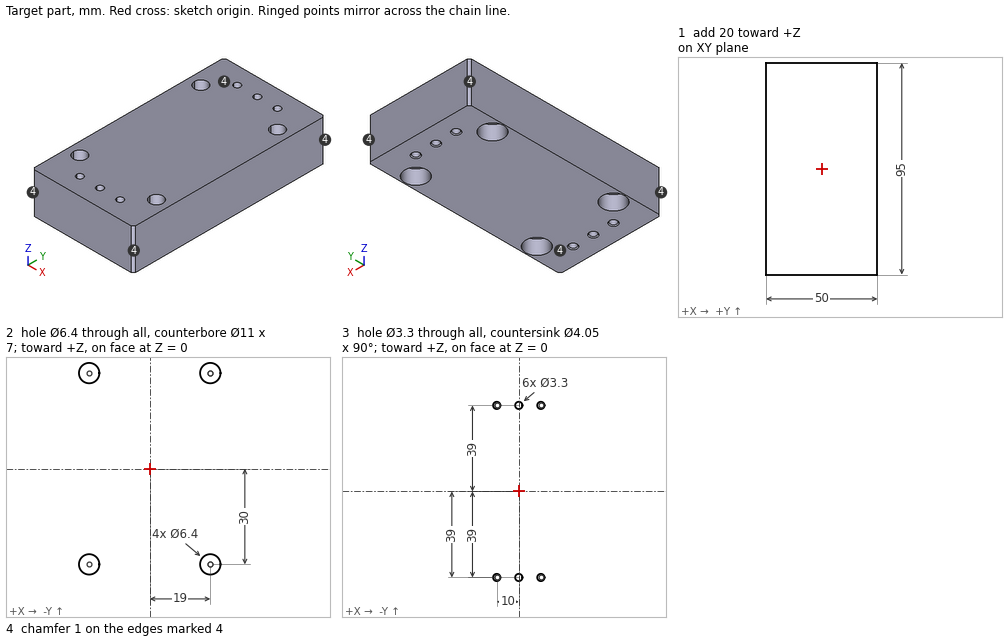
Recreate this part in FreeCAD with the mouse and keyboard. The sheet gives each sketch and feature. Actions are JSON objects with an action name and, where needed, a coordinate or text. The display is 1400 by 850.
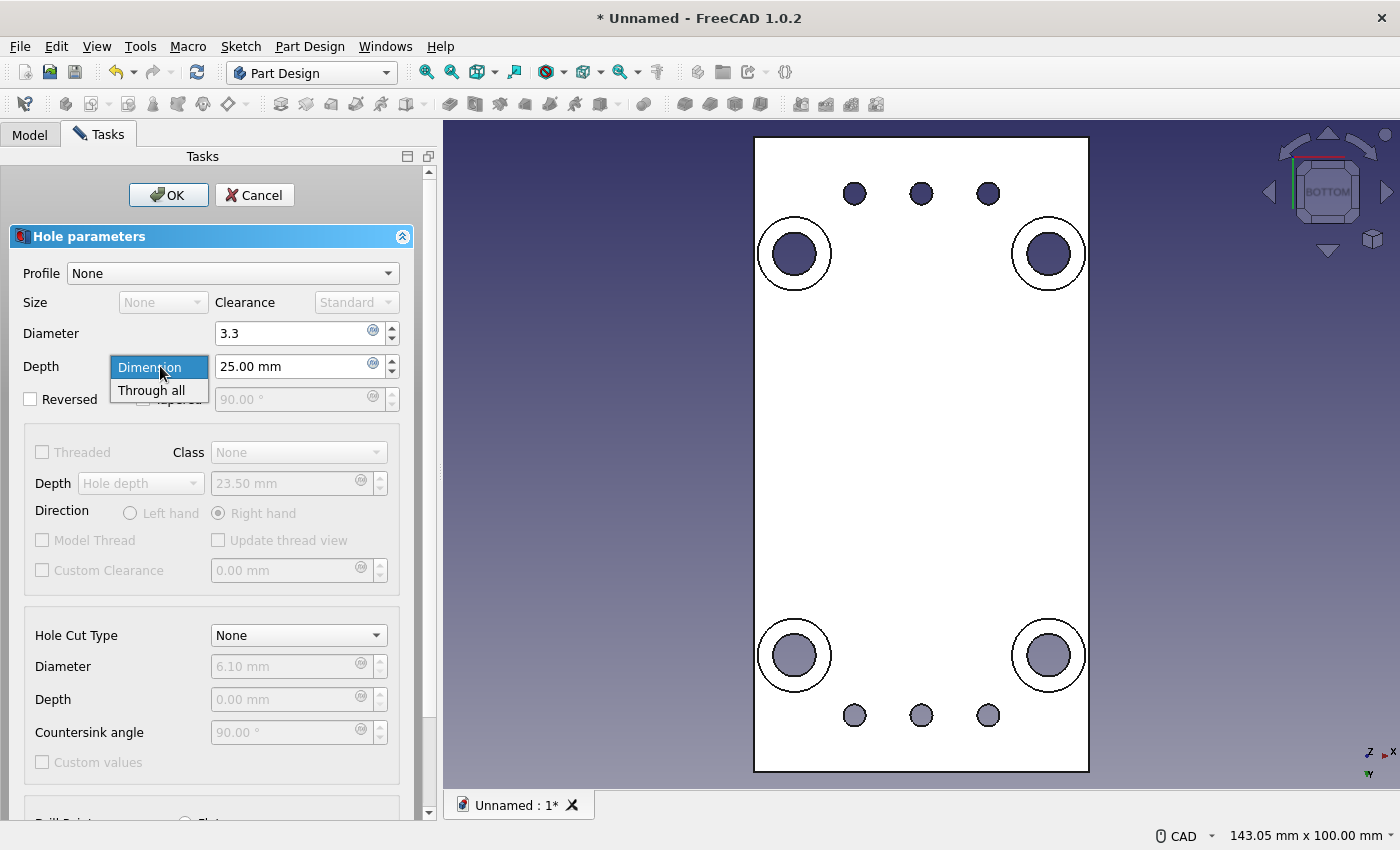
{"action": "left_click", "coordinate": [158, 390]}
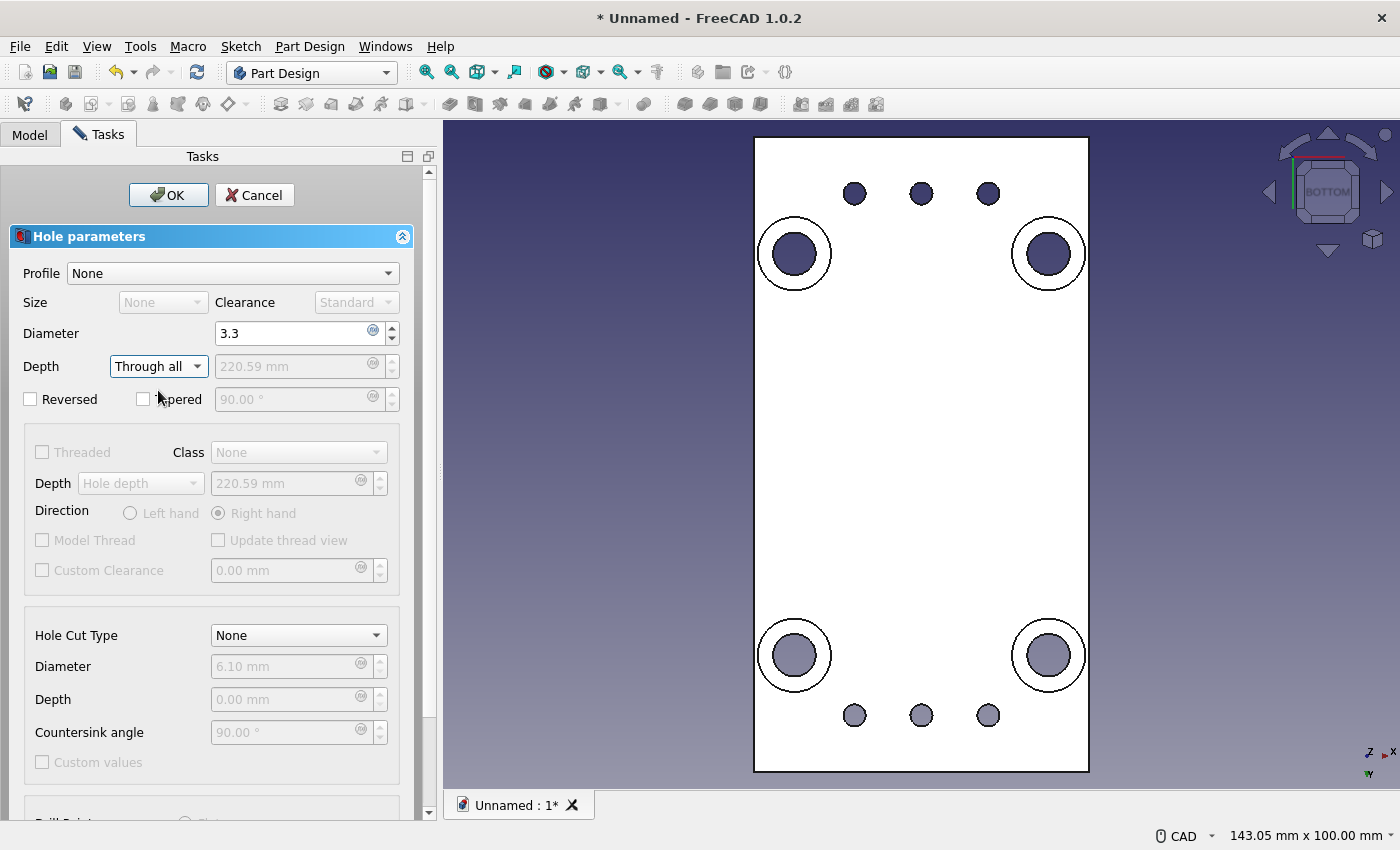
{"action": "left_click", "coordinate": [300, 636]}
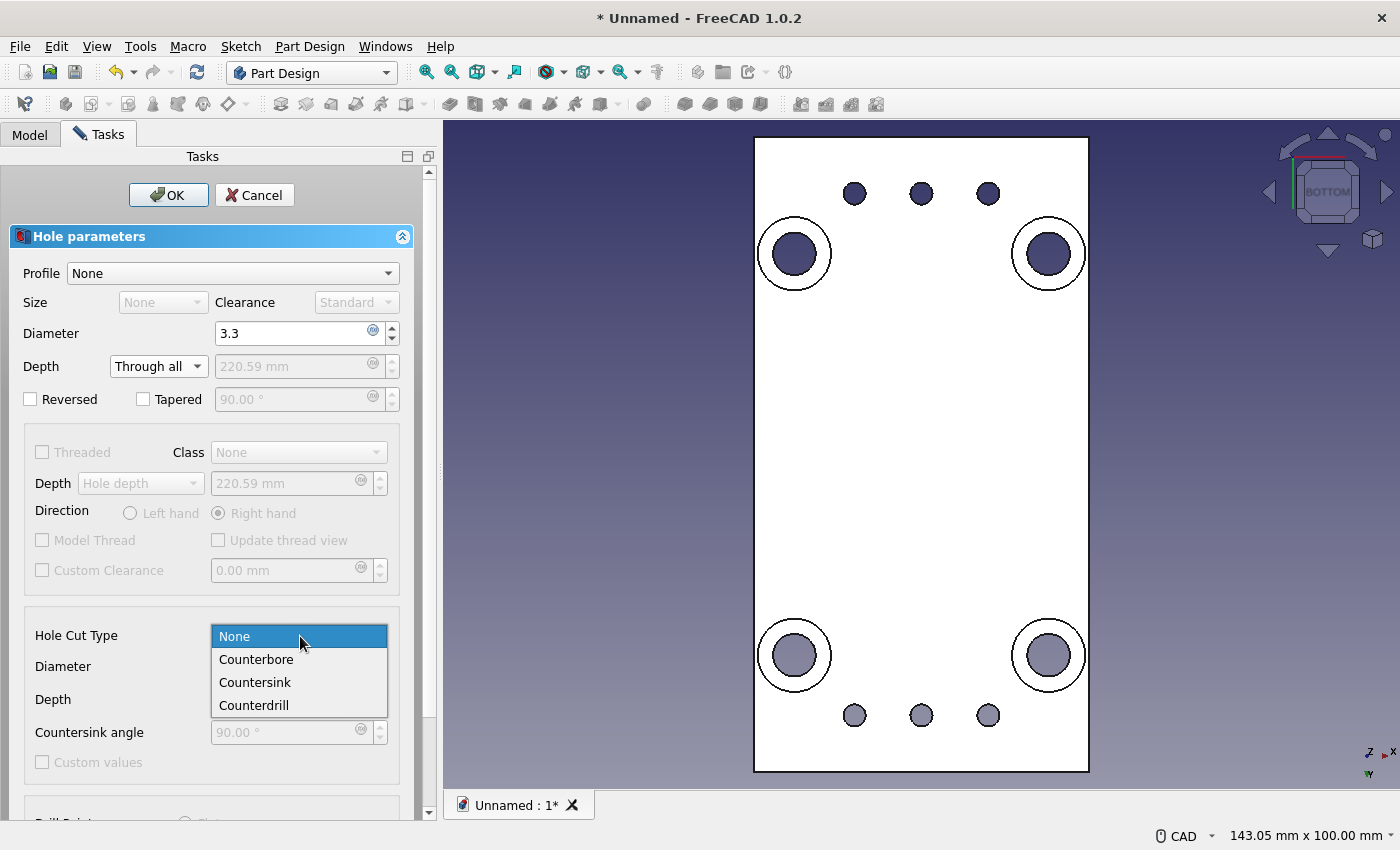
{"action": "left_click", "coordinate": [298, 682]}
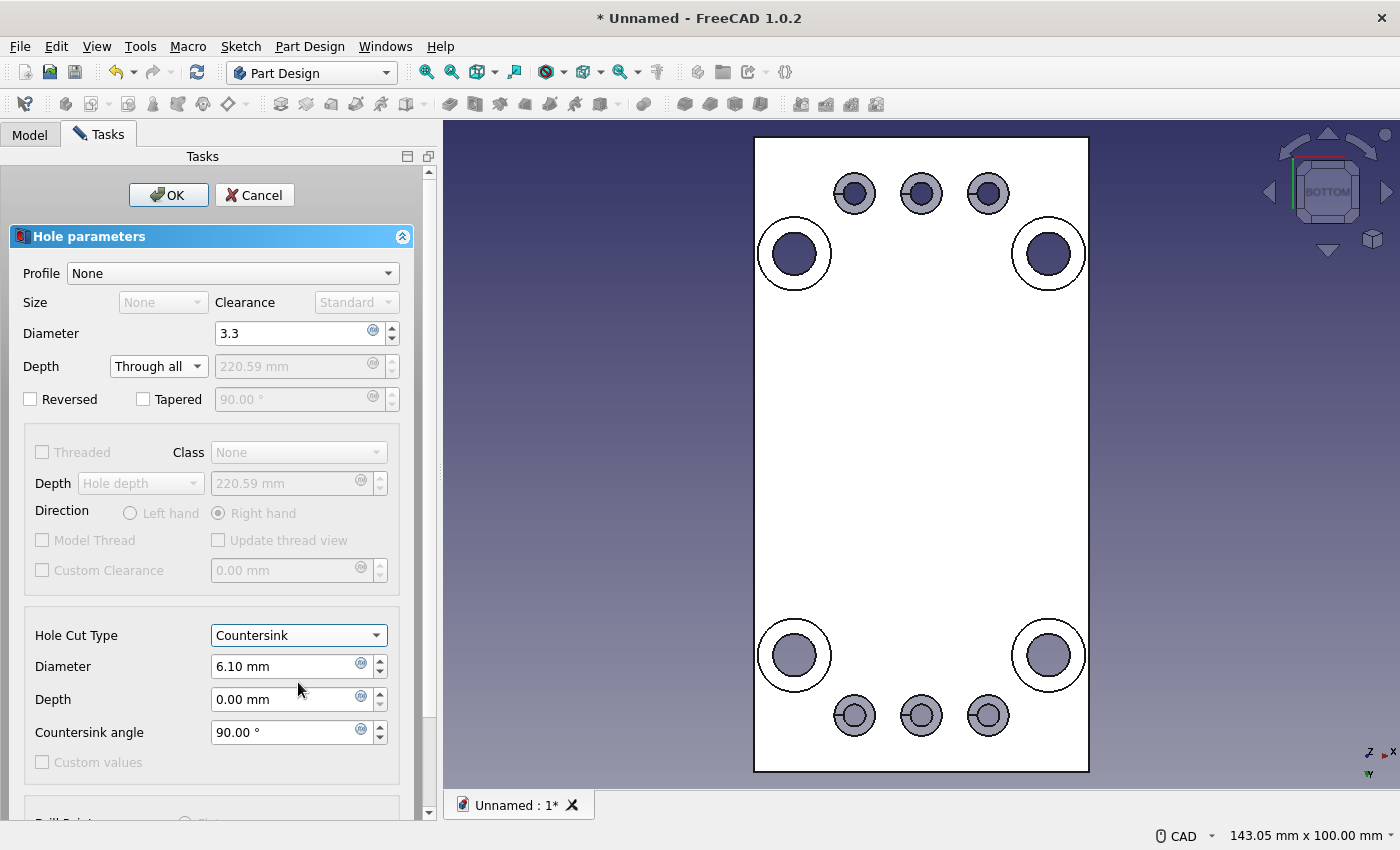
{"action": "triple_click", "coordinate": [292, 666]}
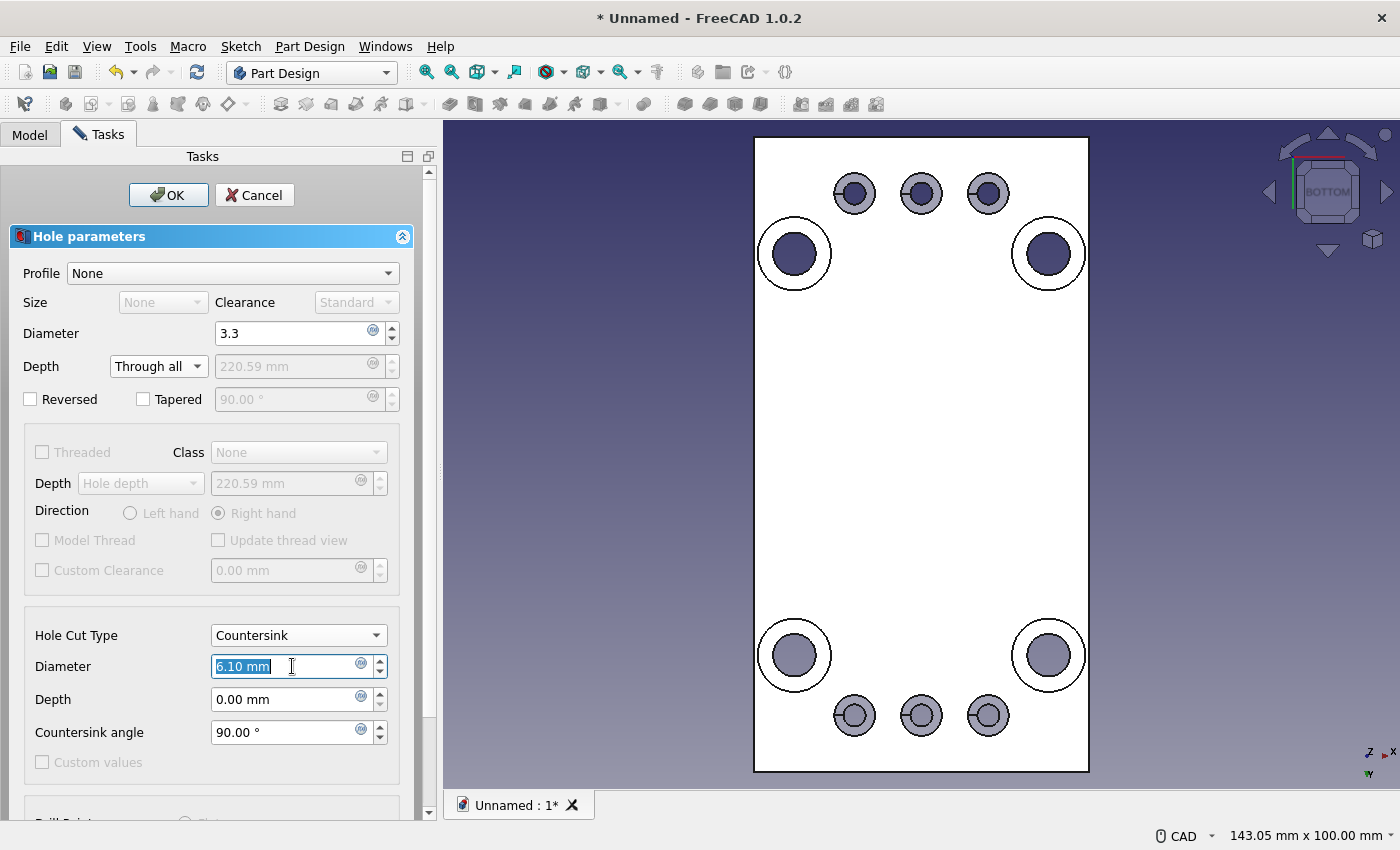
{"action": "type", "text": "4.05"}
{"action": "key", "text": "Tab"}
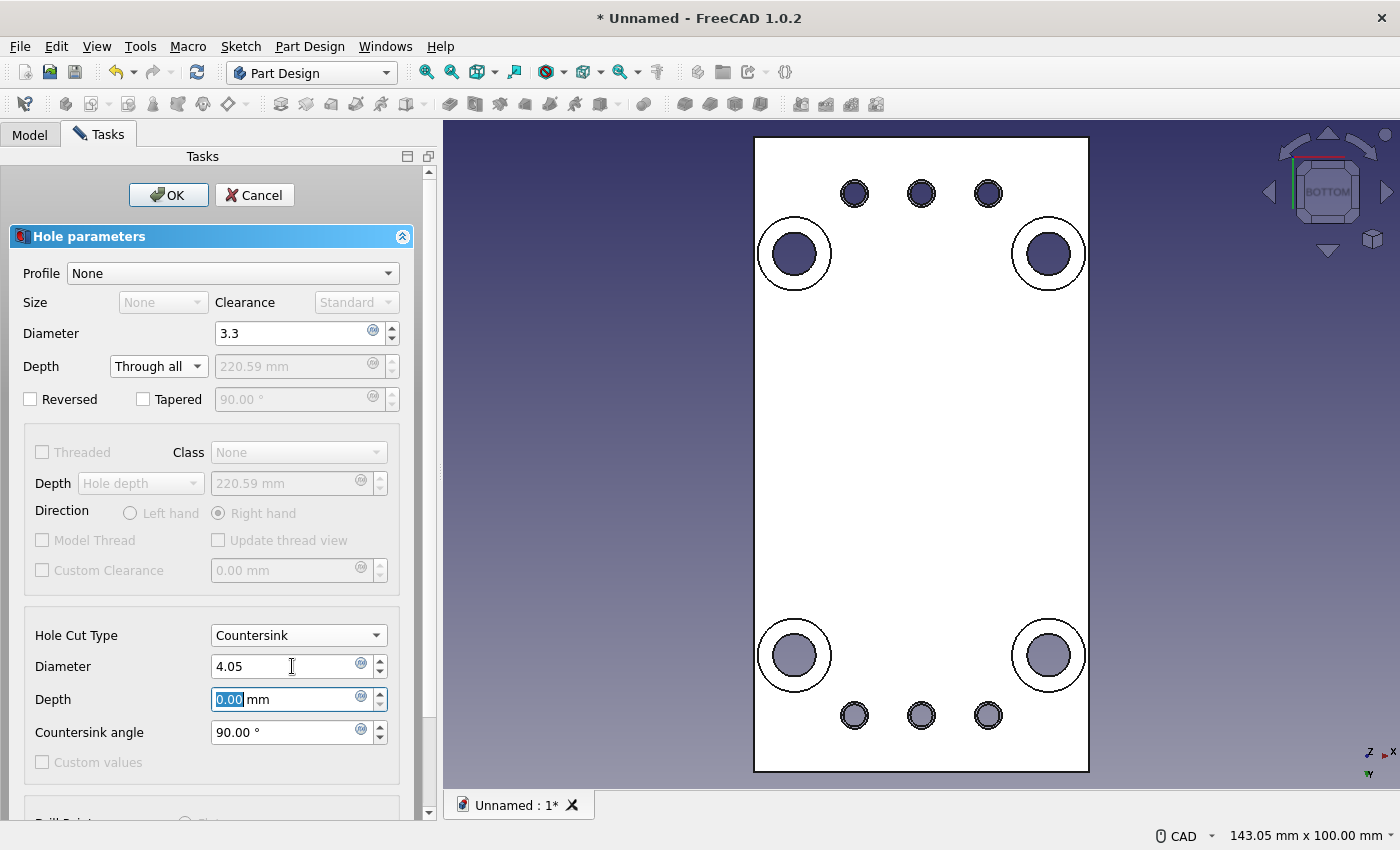
{"action": "left_click", "coordinate": [169, 195]}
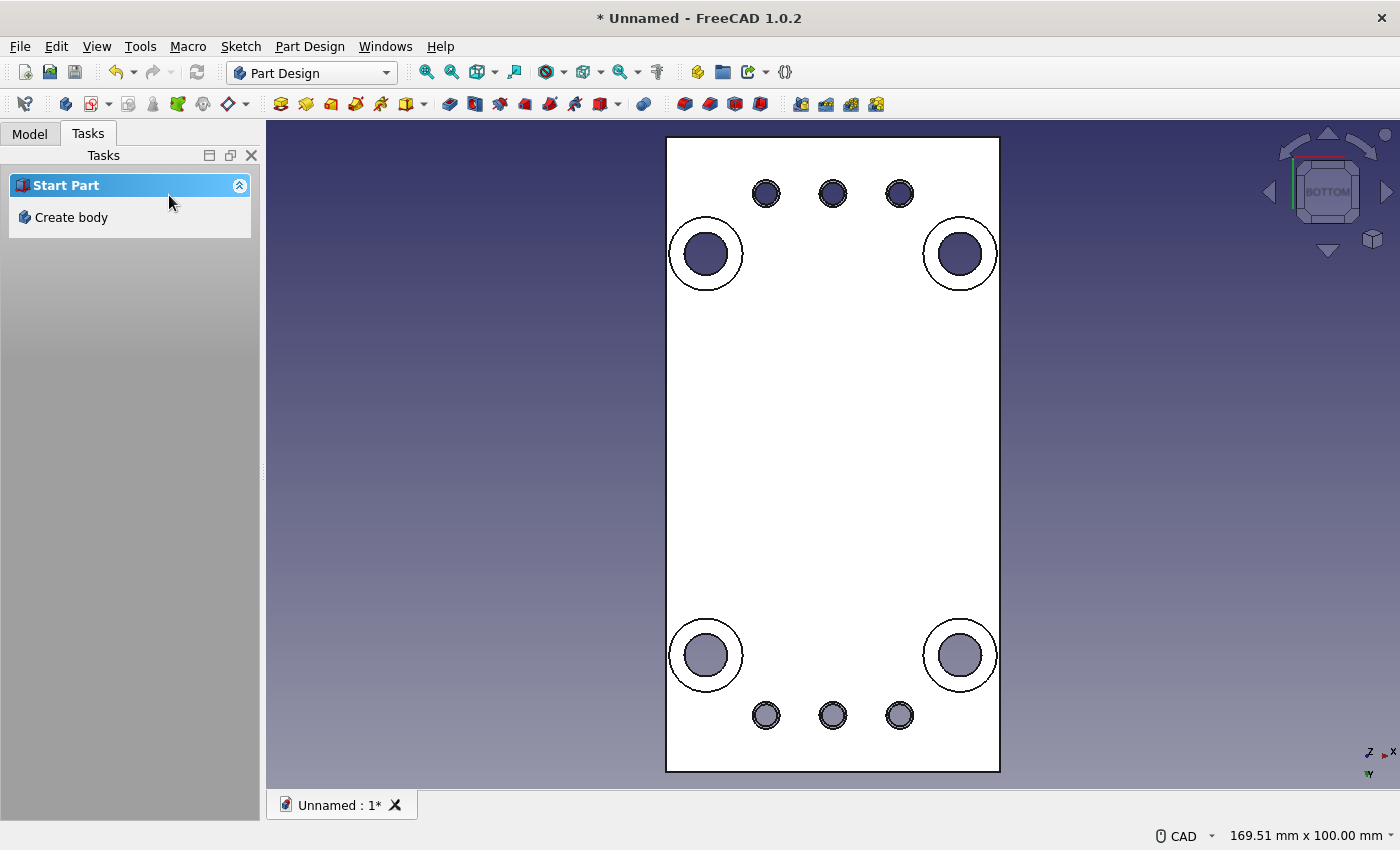
{"action": "key", "text": "0"}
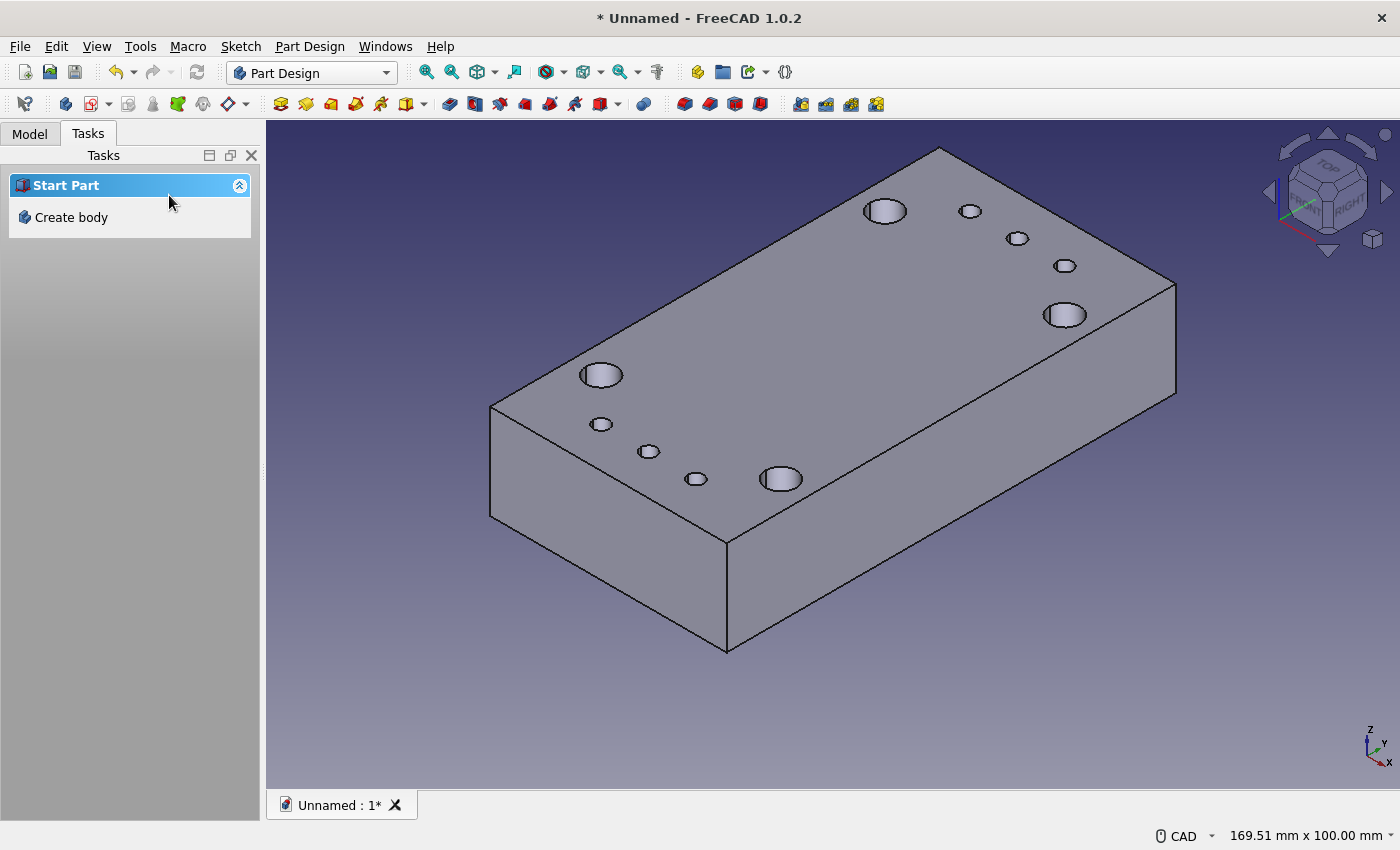
{"action": "left_click", "coordinate": [727, 597]}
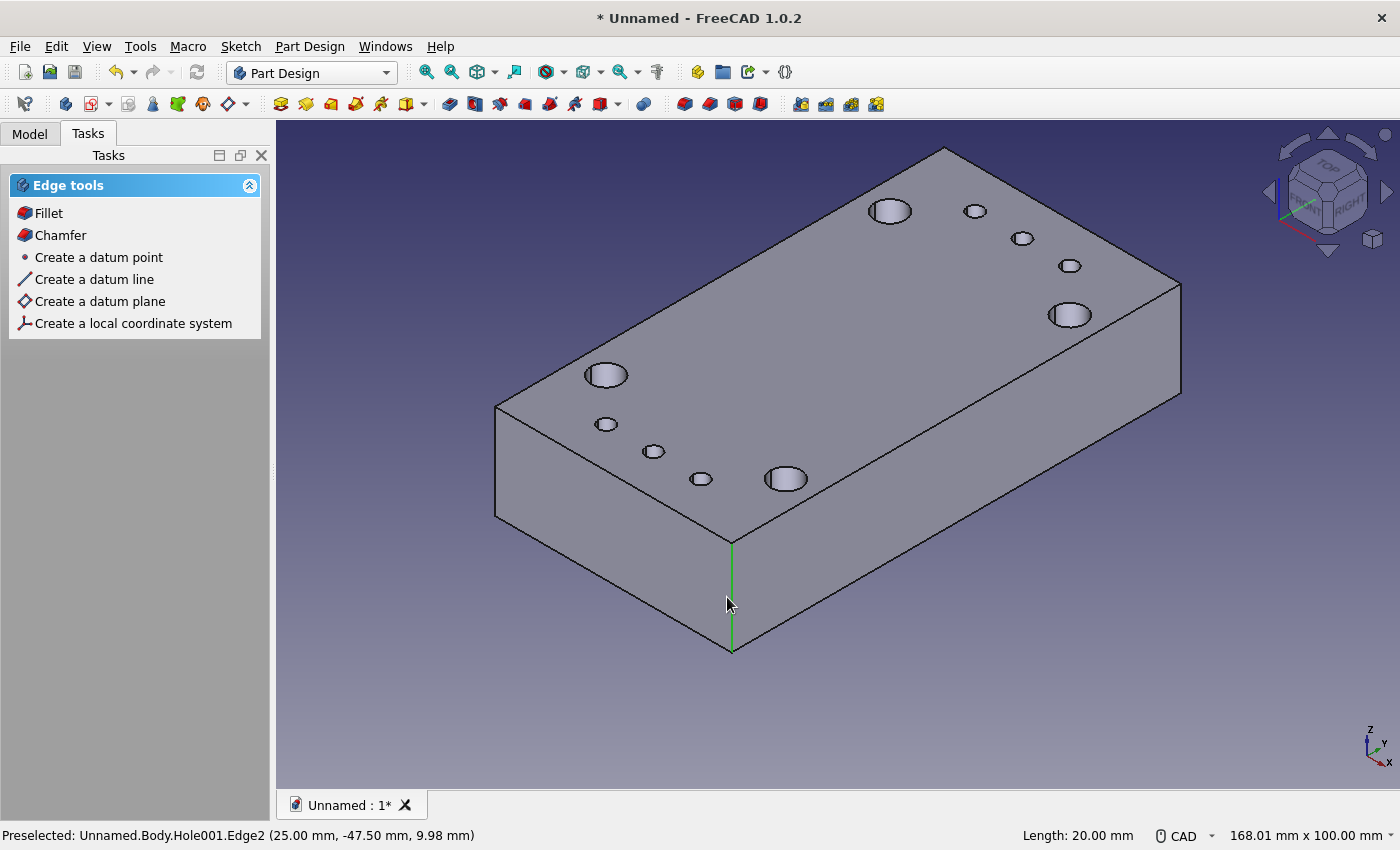
{"action": "key", "text": "2"}